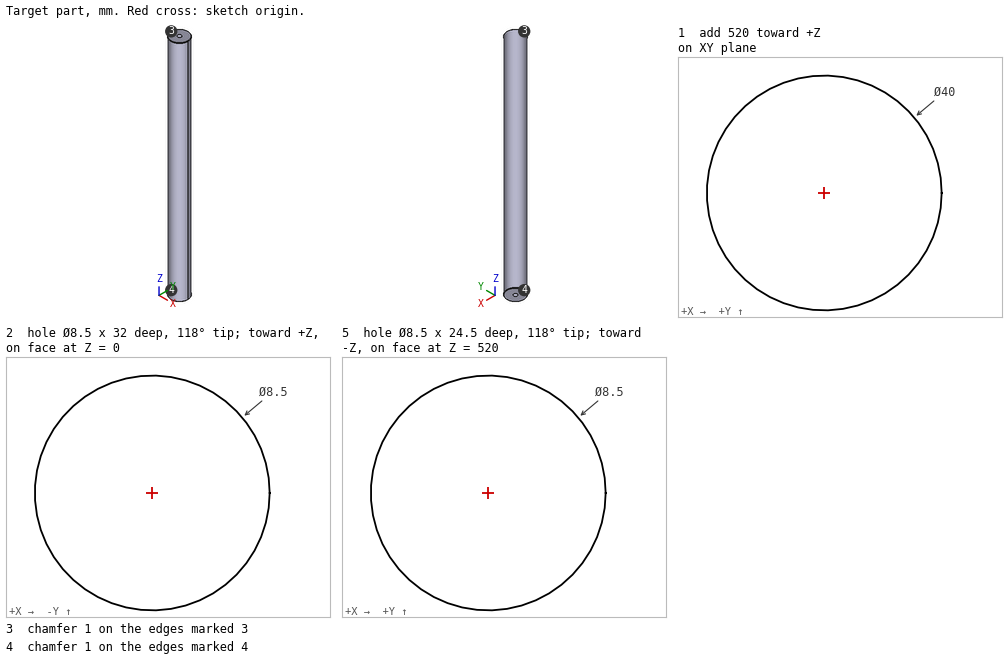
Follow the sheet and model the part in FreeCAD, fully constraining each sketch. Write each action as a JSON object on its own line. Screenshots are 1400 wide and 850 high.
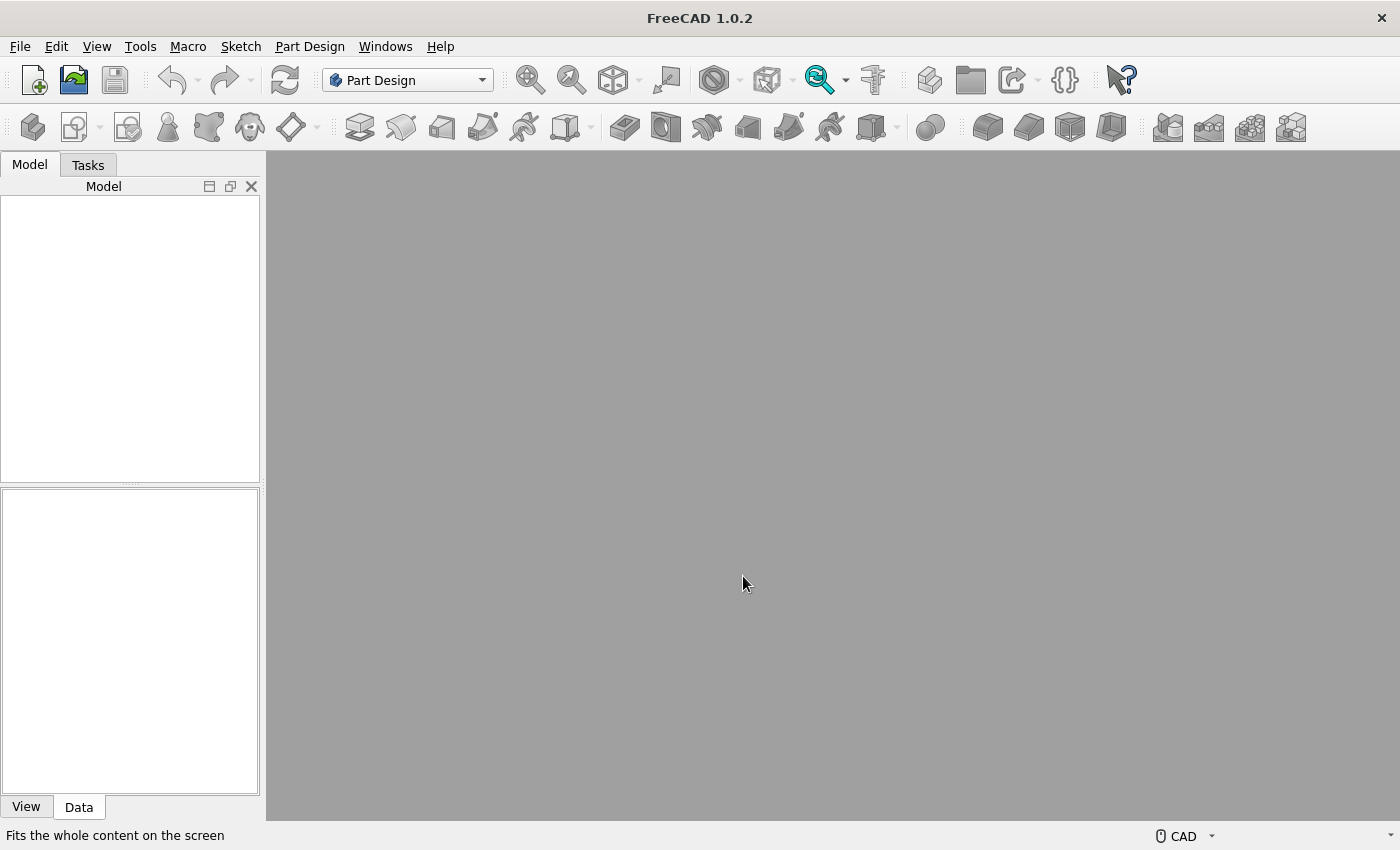
{"action": "left_click", "coordinate": [33, 80]}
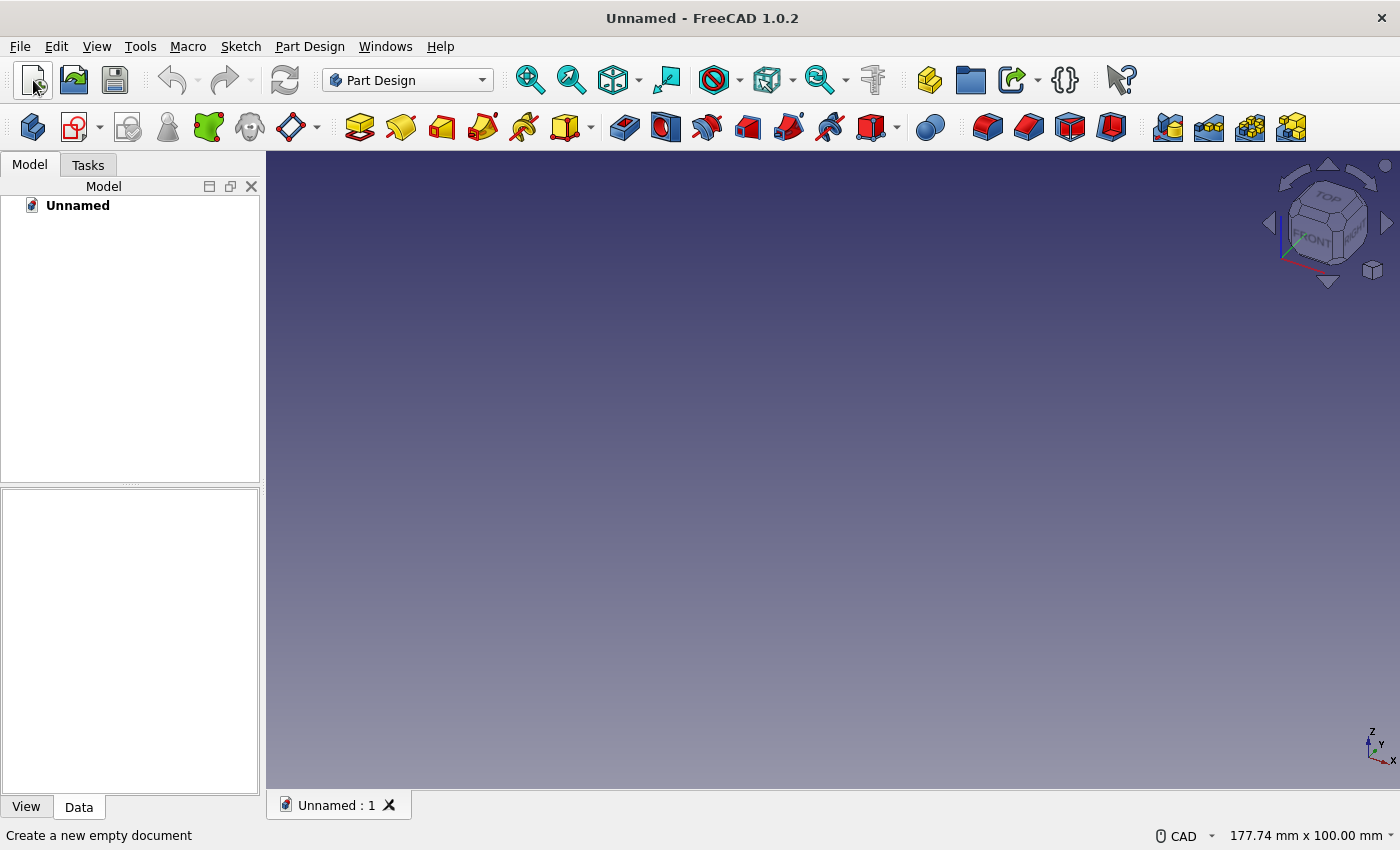
{"action": "left_click", "coordinate": [74, 128]}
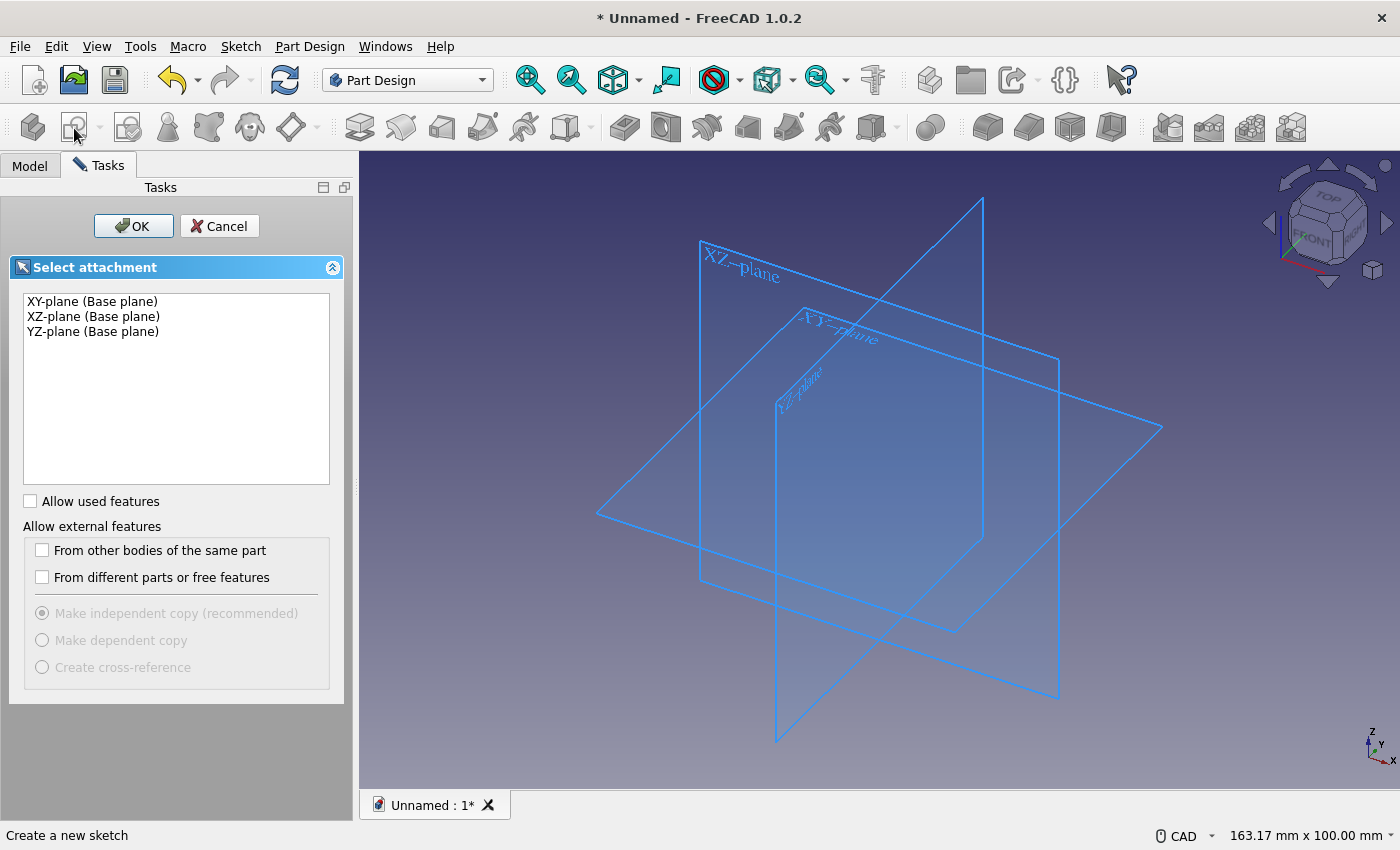
{"action": "left_click", "coordinate": [84, 302]}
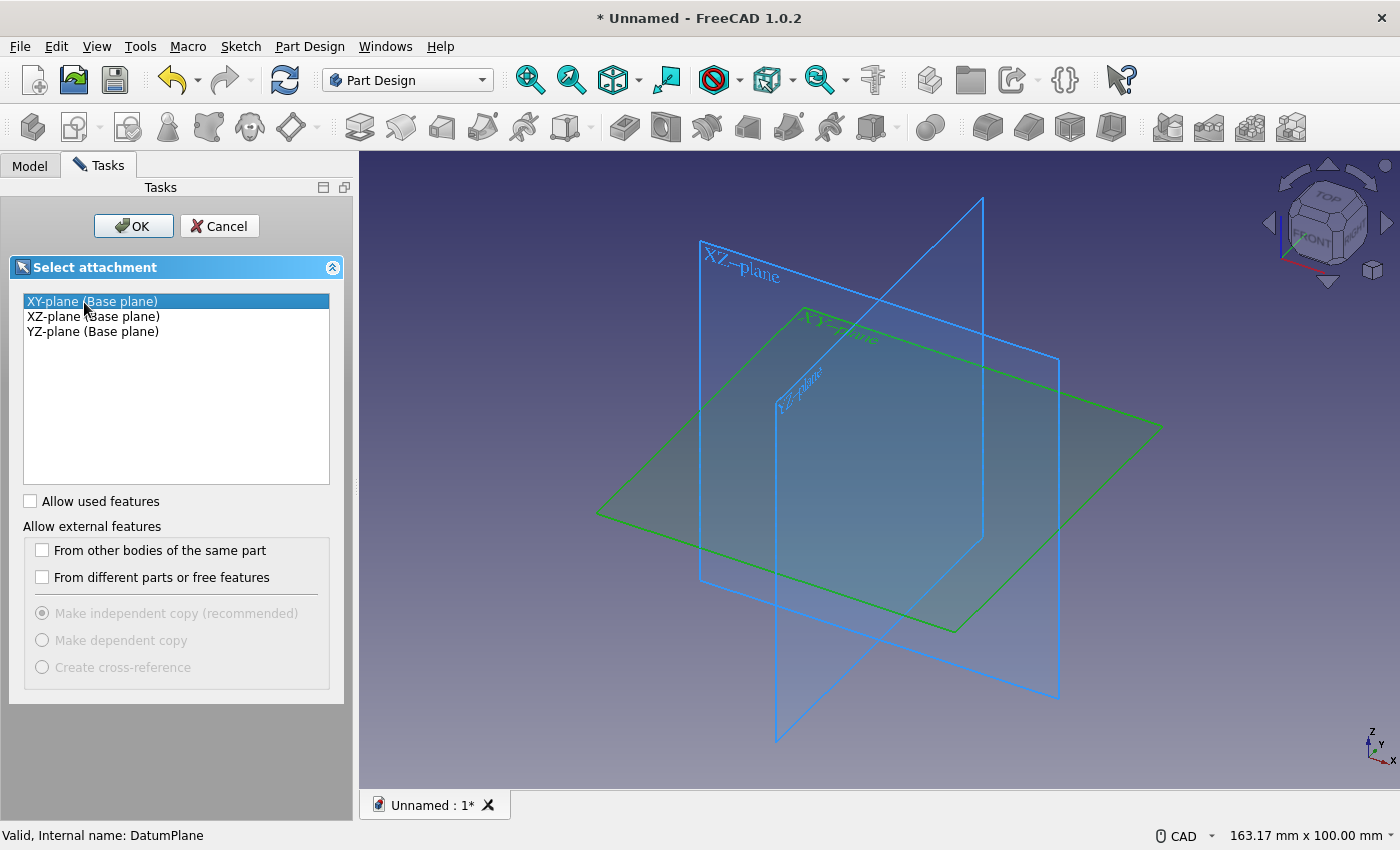
{"action": "left_click", "coordinate": [134, 226]}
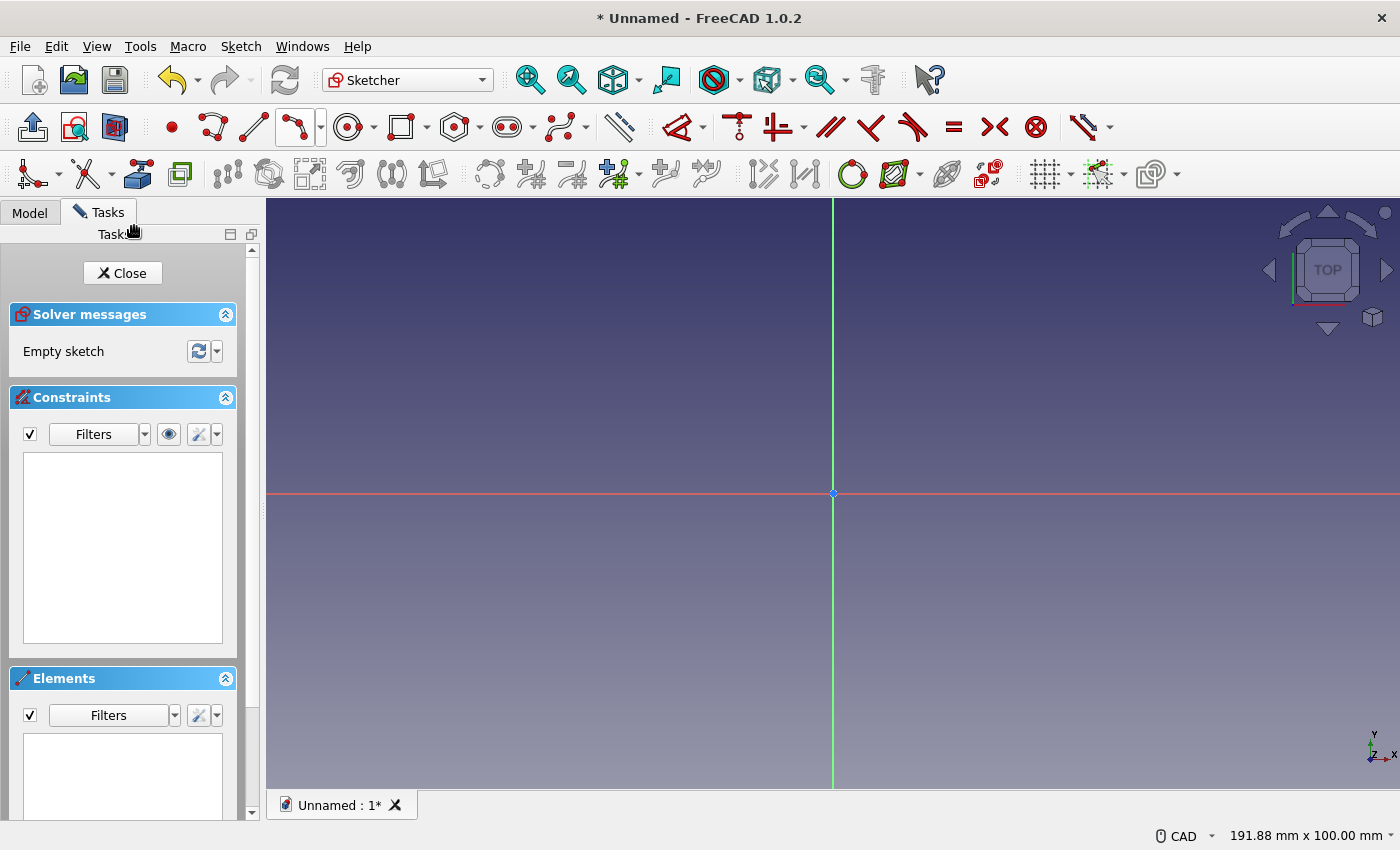
{"action": "scroll", "coordinate": [972, 493], "scroll_direction": "up", "scroll_amount": 2}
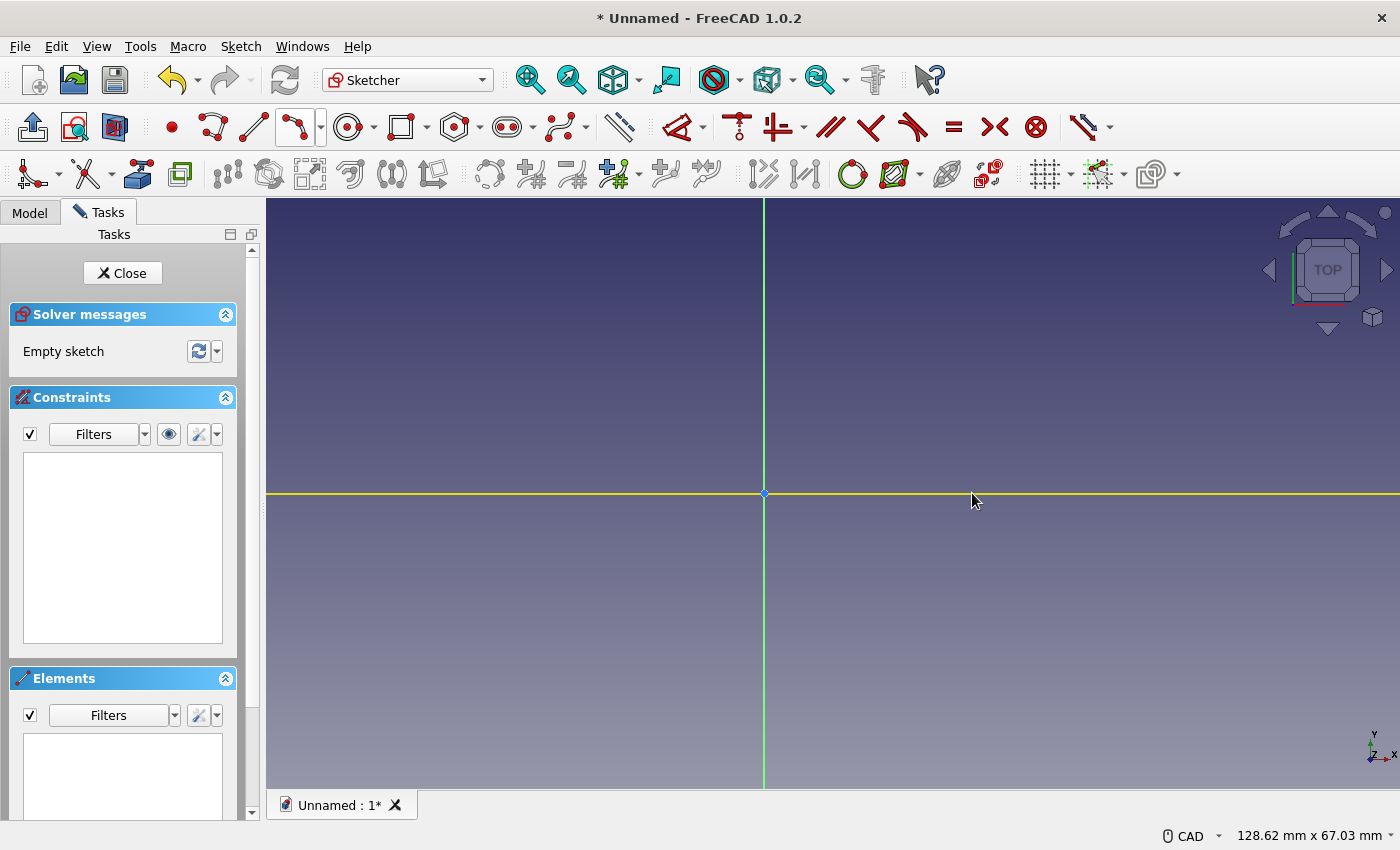
{"action": "left_click", "coordinate": [348, 128]}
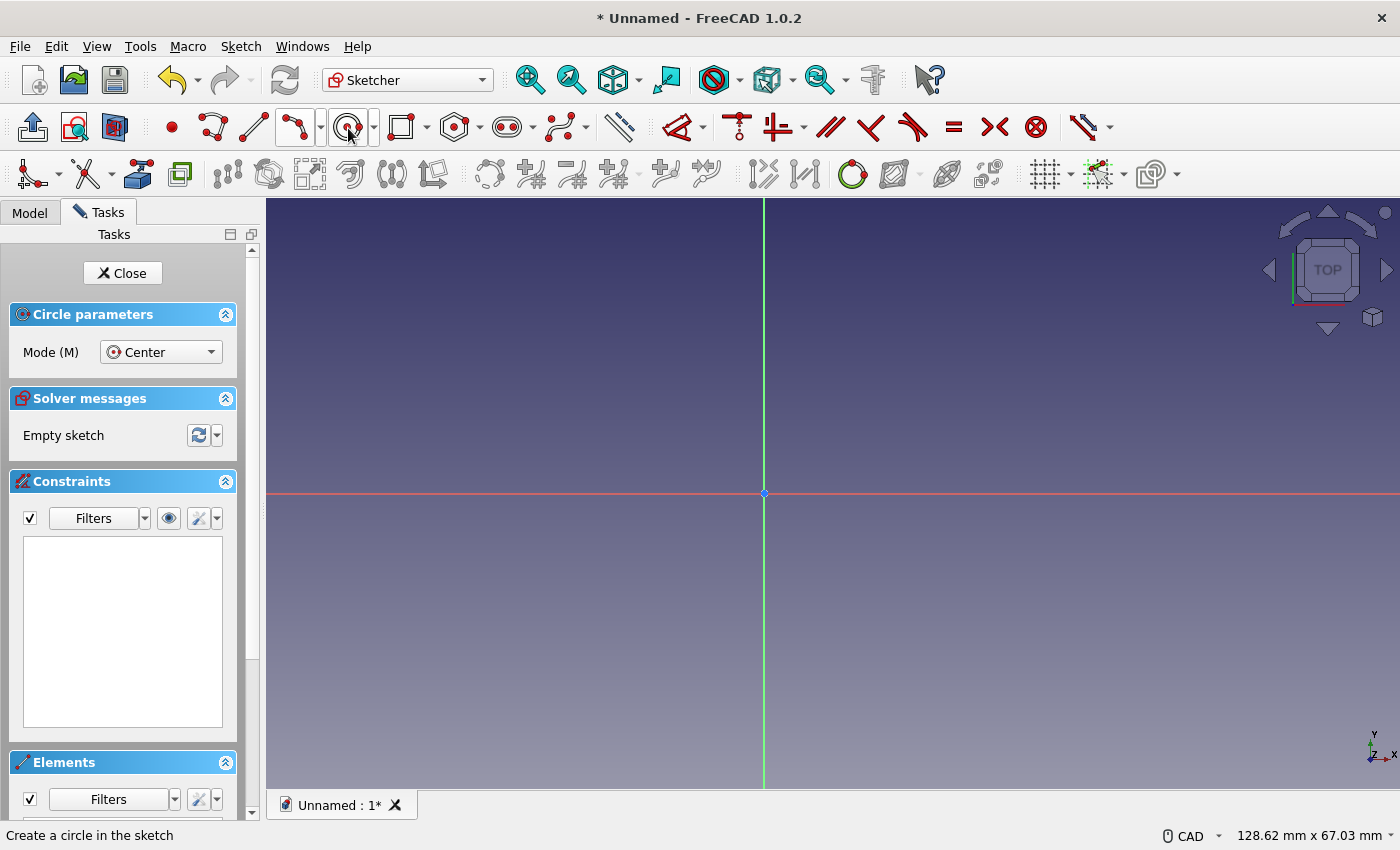
{"action": "left_click", "coordinate": [764, 494]}
{"action": "left_click", "coordinate": [889, 369]}
{"action": "key", "text": "Escape"}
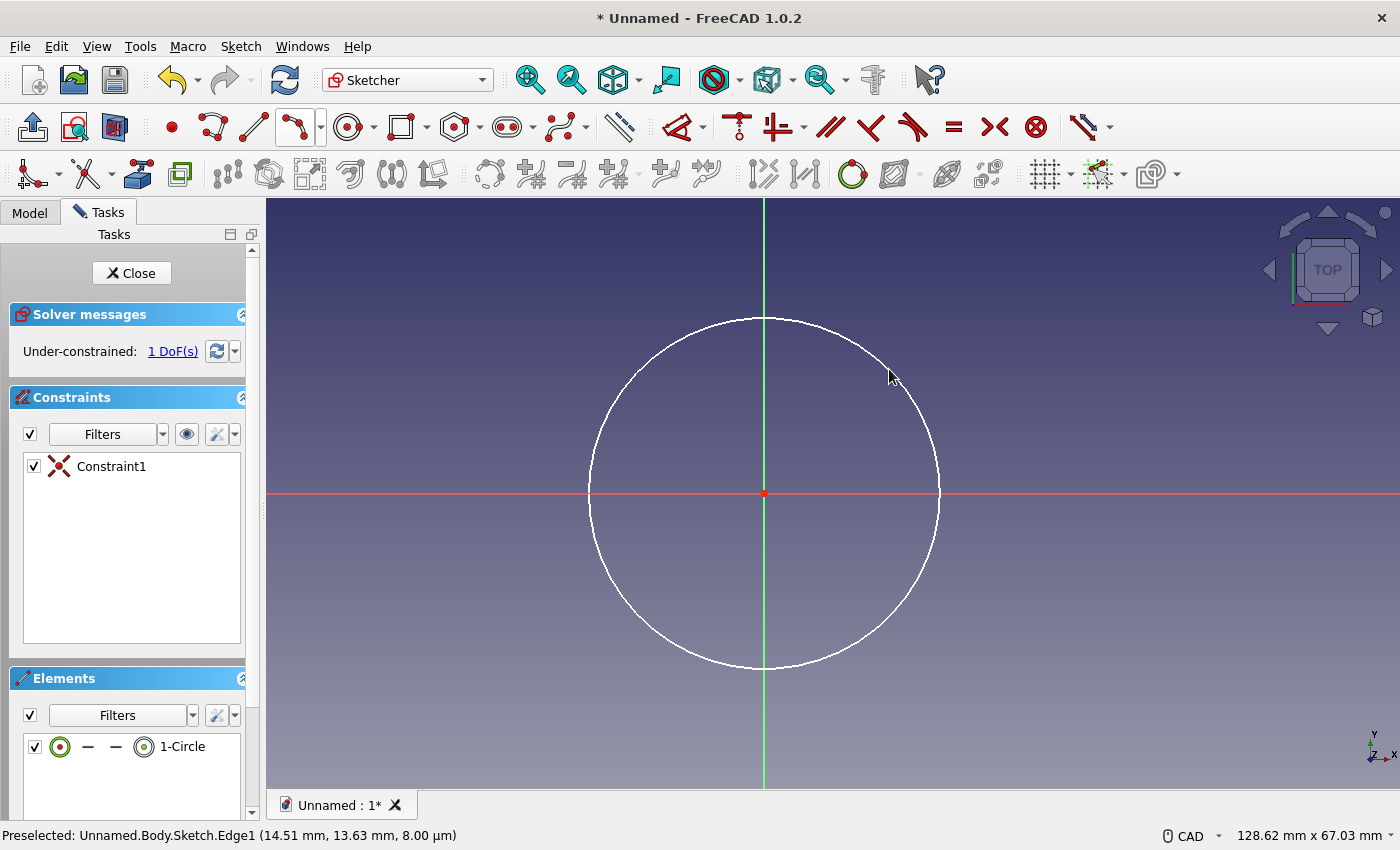
{"action": "left_click", "coordinate": [676, 128]}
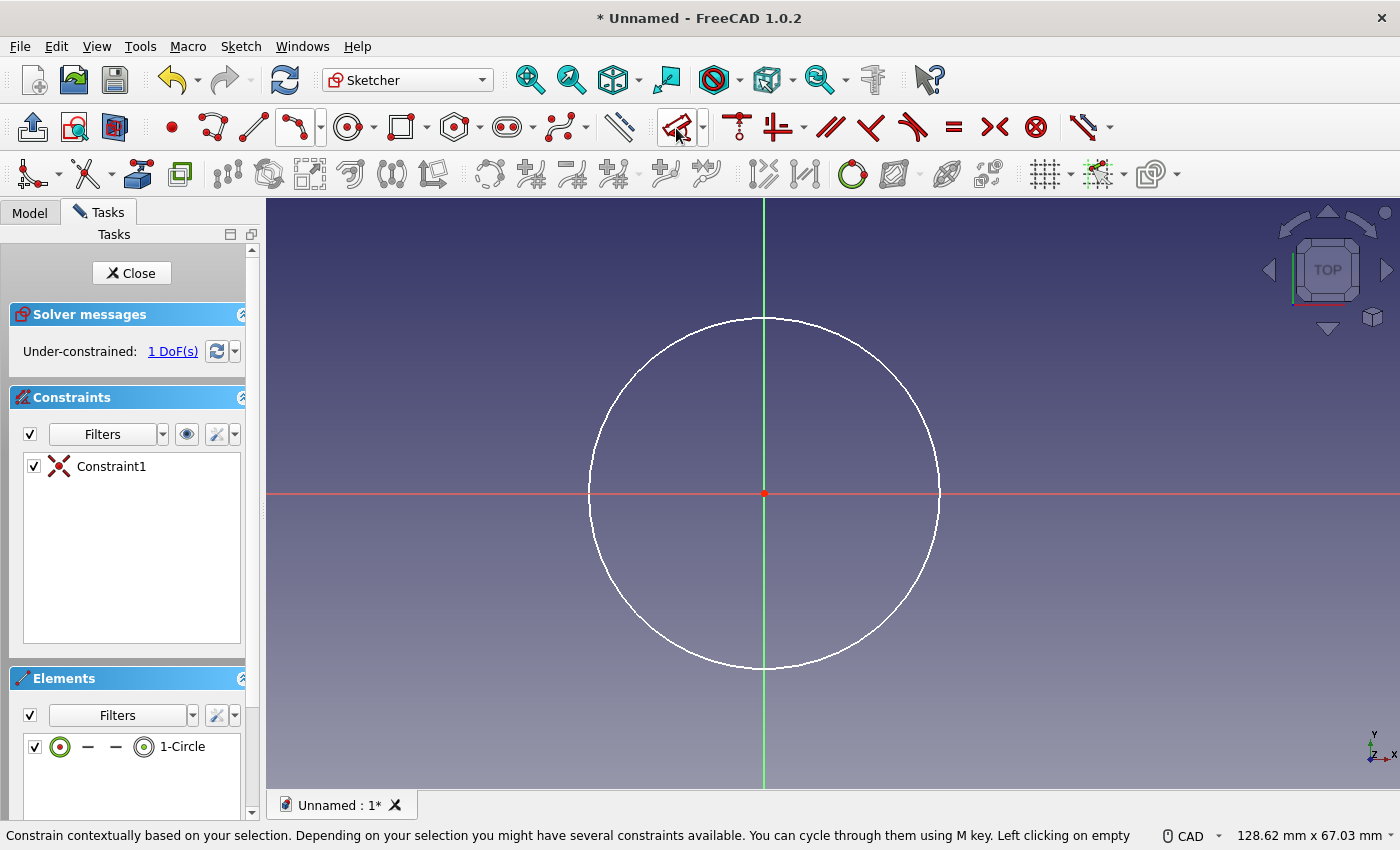
{"action": "left_click", "coordinate": [888, 369]}
{"action": "left_click", "coordinate": [911, 346]}